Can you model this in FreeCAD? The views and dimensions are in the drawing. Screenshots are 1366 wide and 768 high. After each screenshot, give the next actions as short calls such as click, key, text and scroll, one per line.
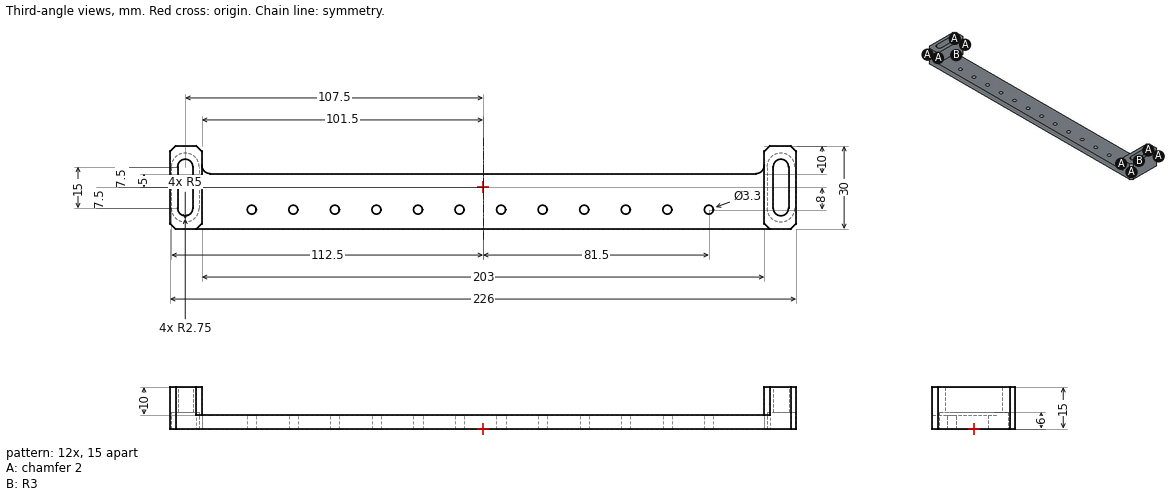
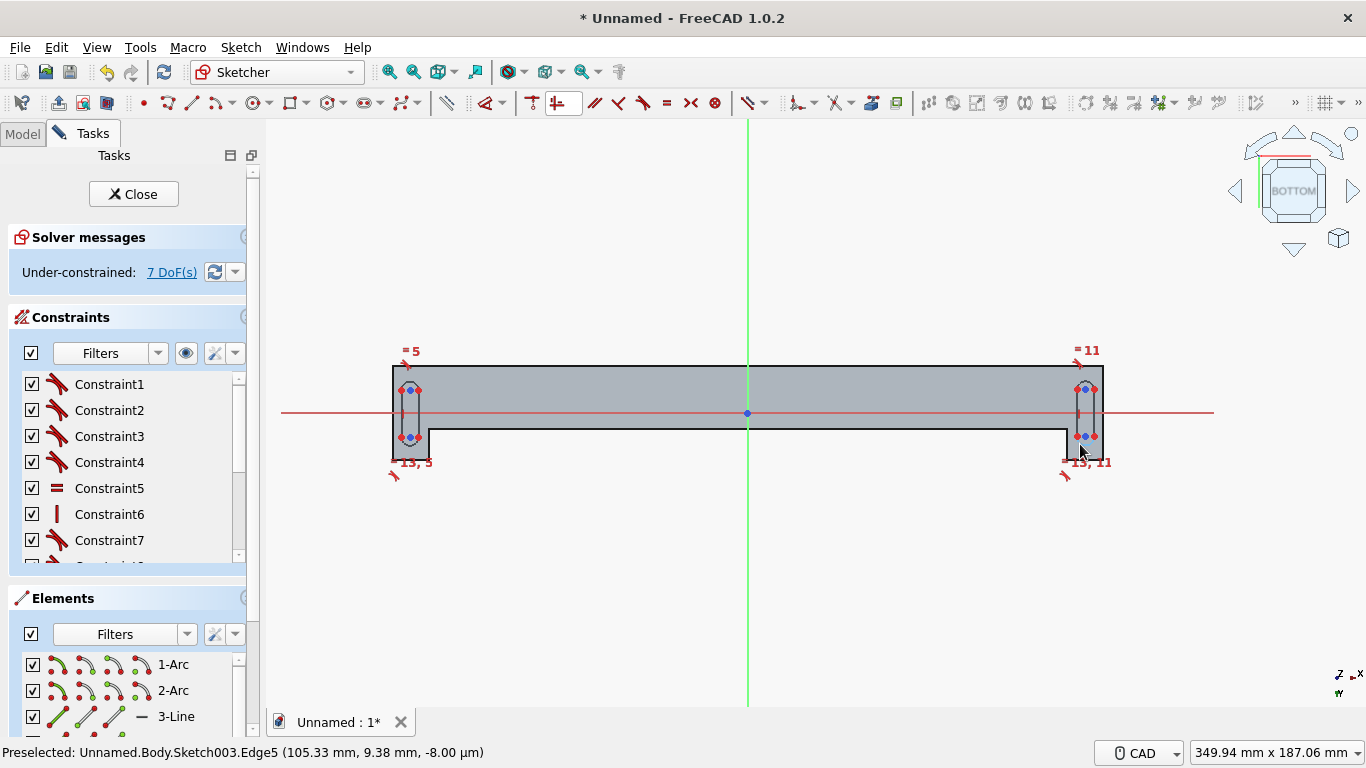
scroll(410, 437, up, 2)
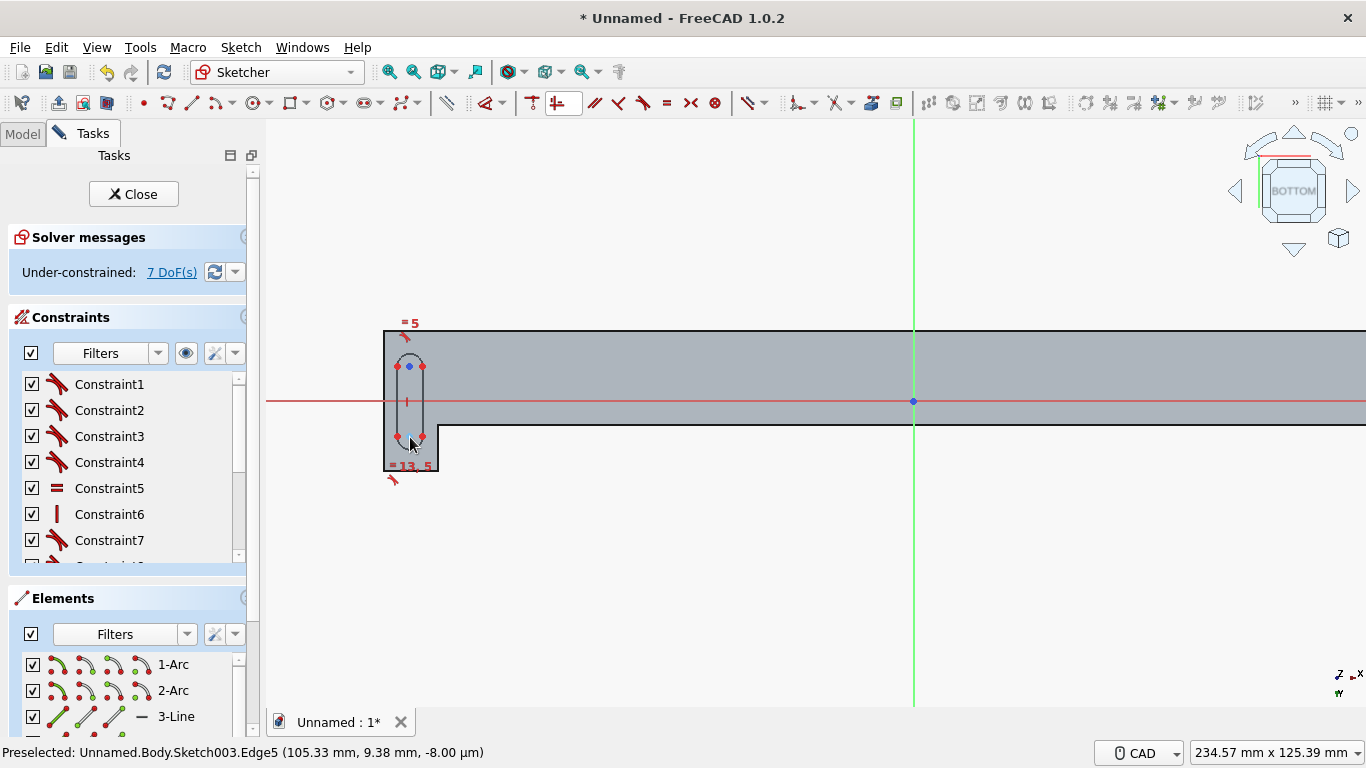
click(410, 437)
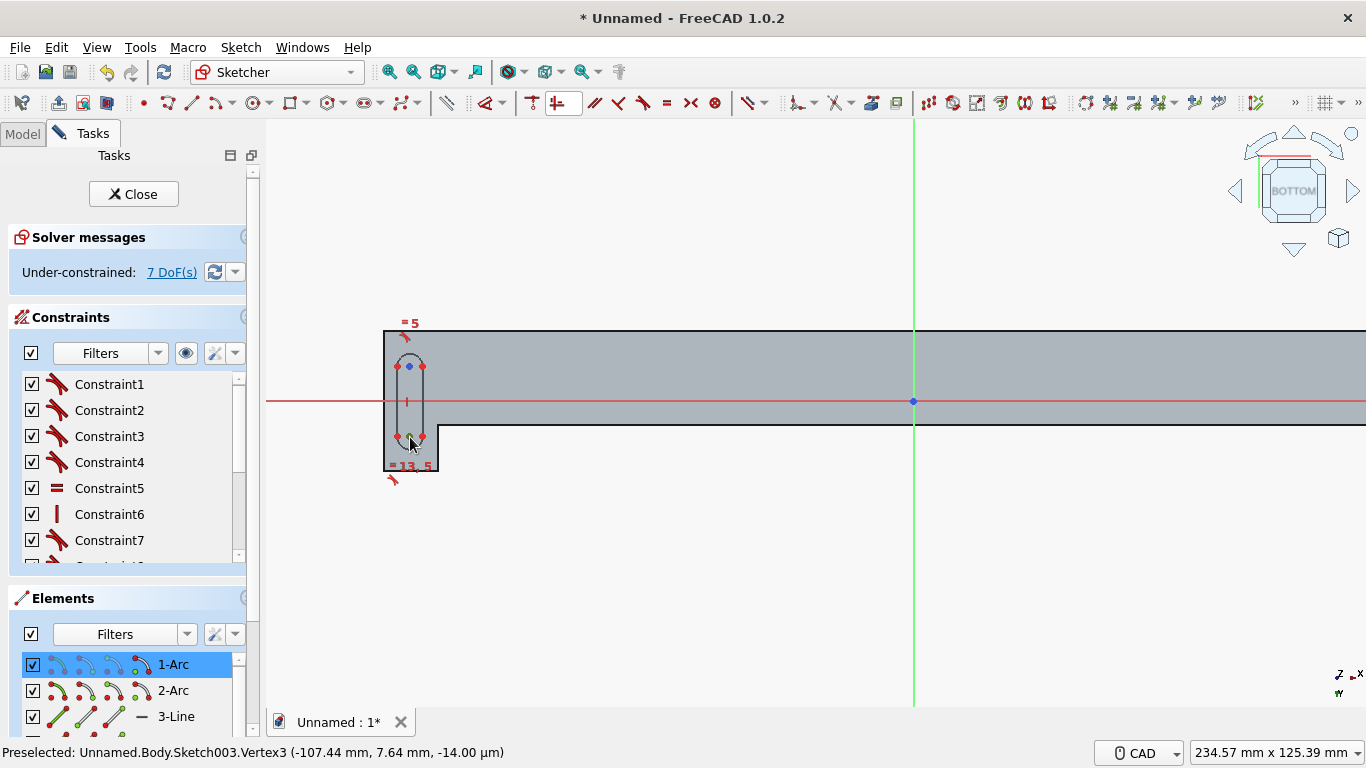
scroll(409, 437, down, 2)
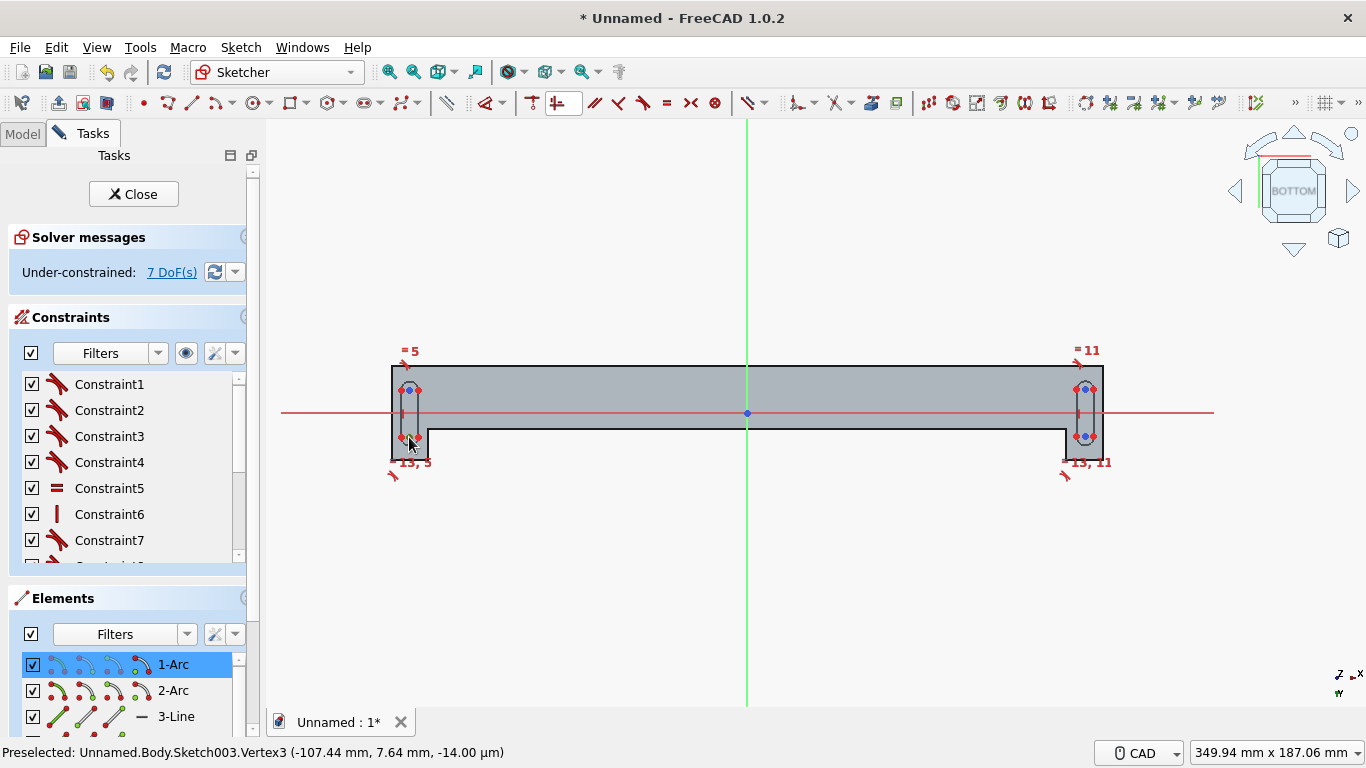
scroll(1085, 437, up, 2)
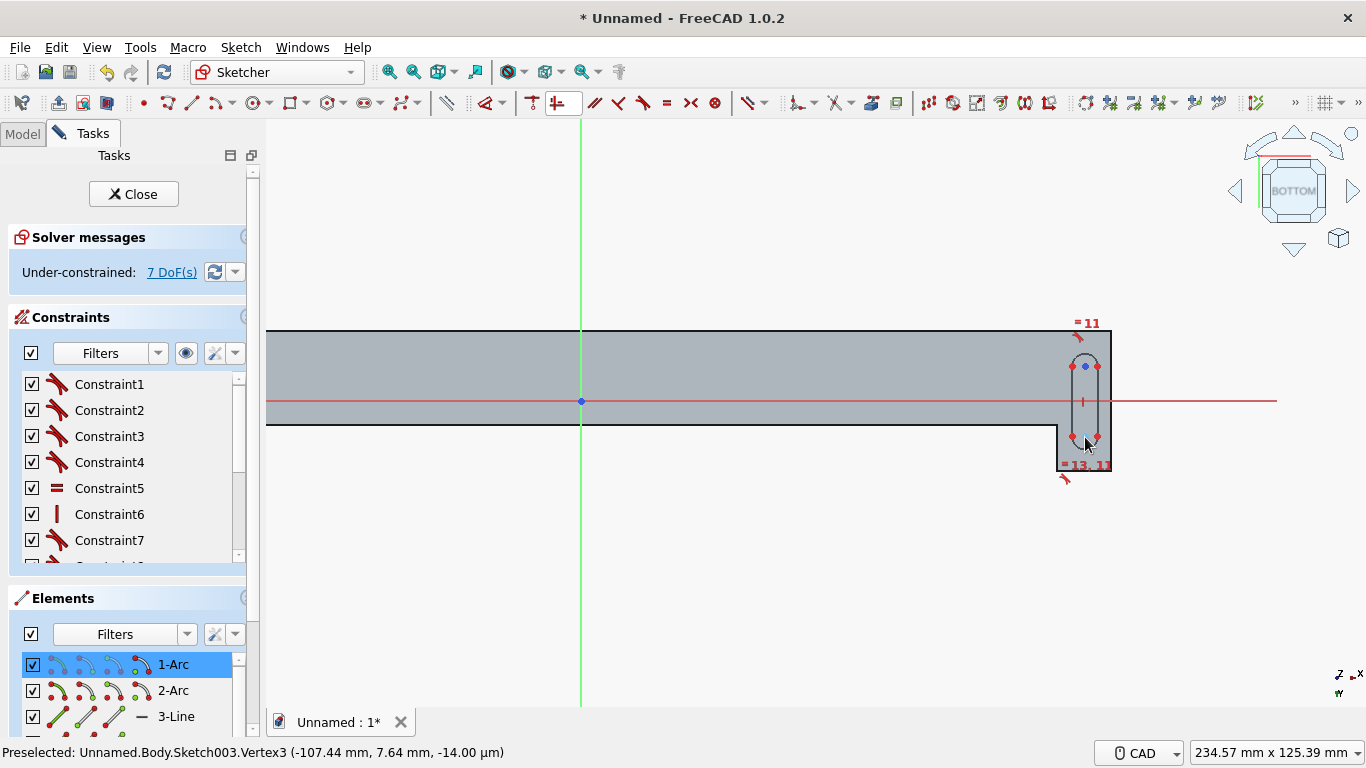
click(1085, 437)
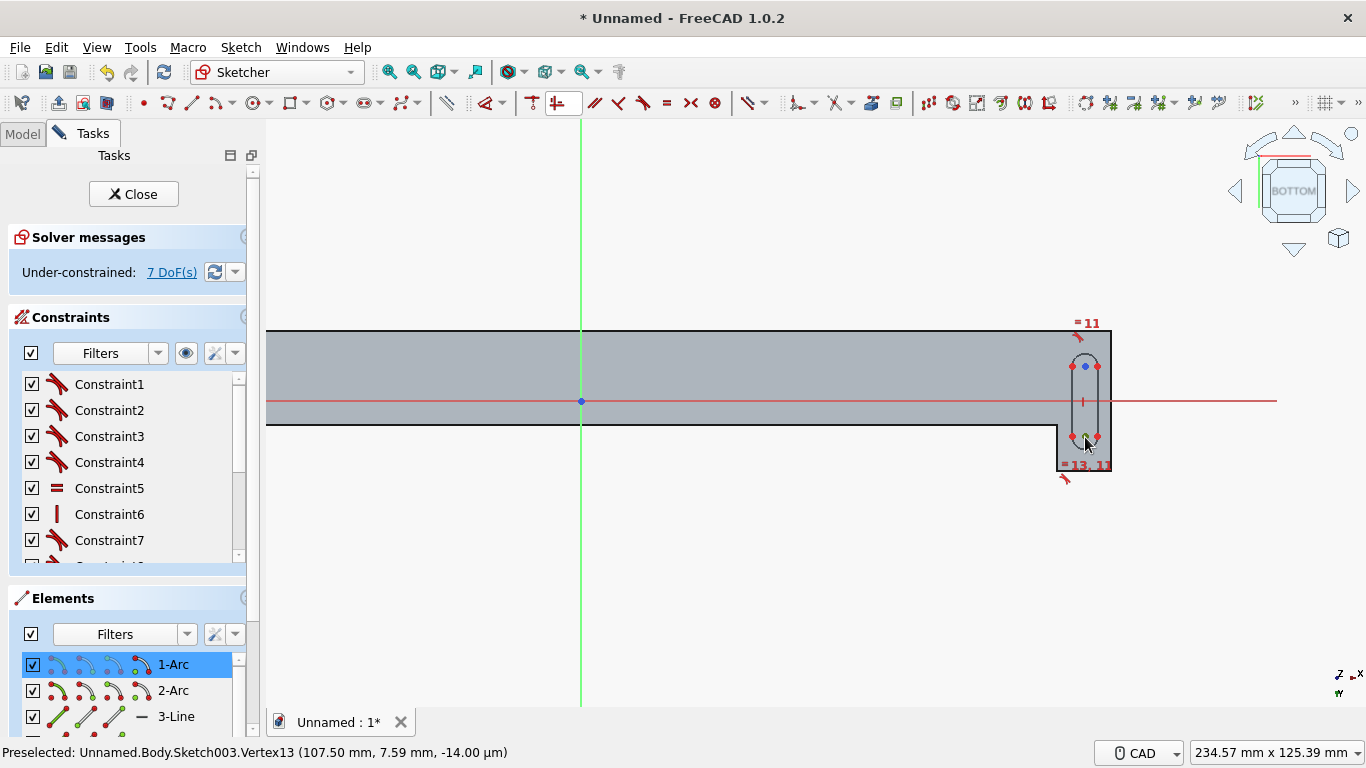
click(581, 641)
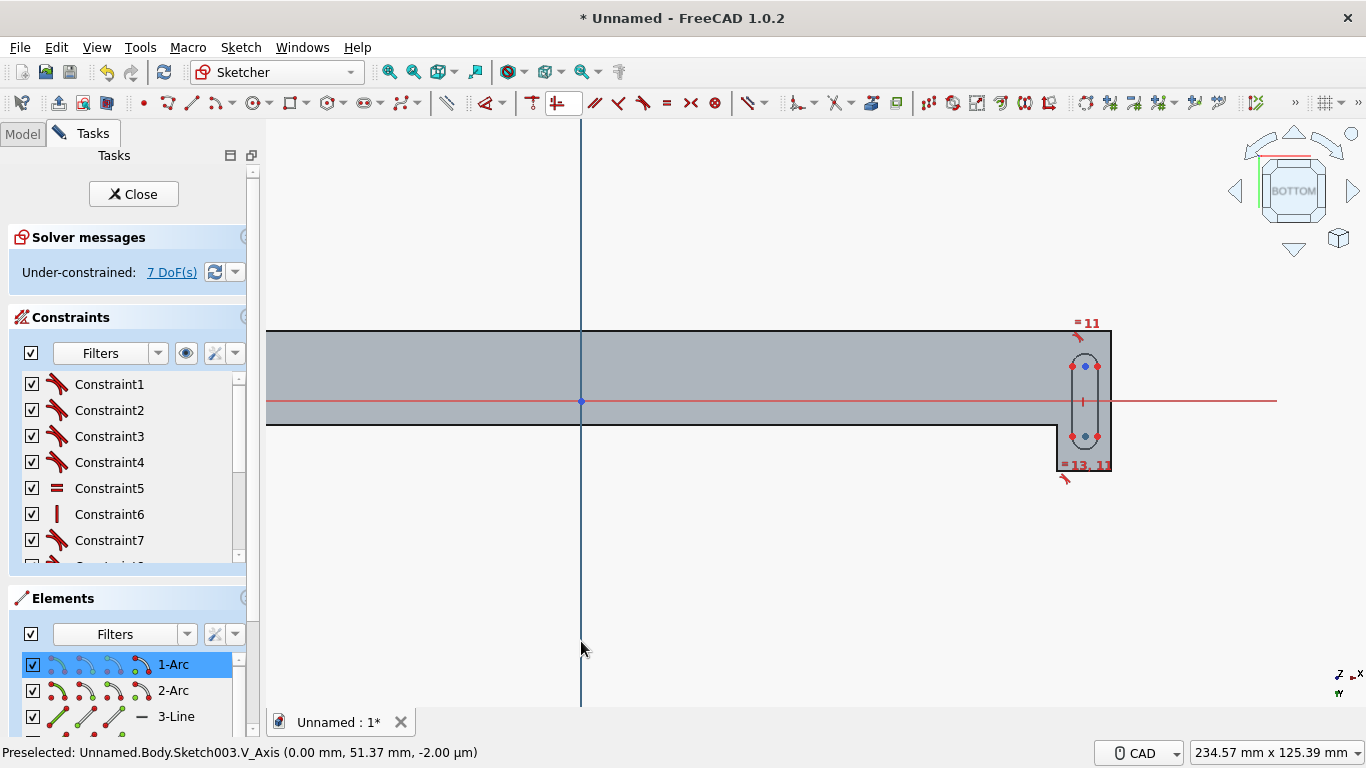
key(s)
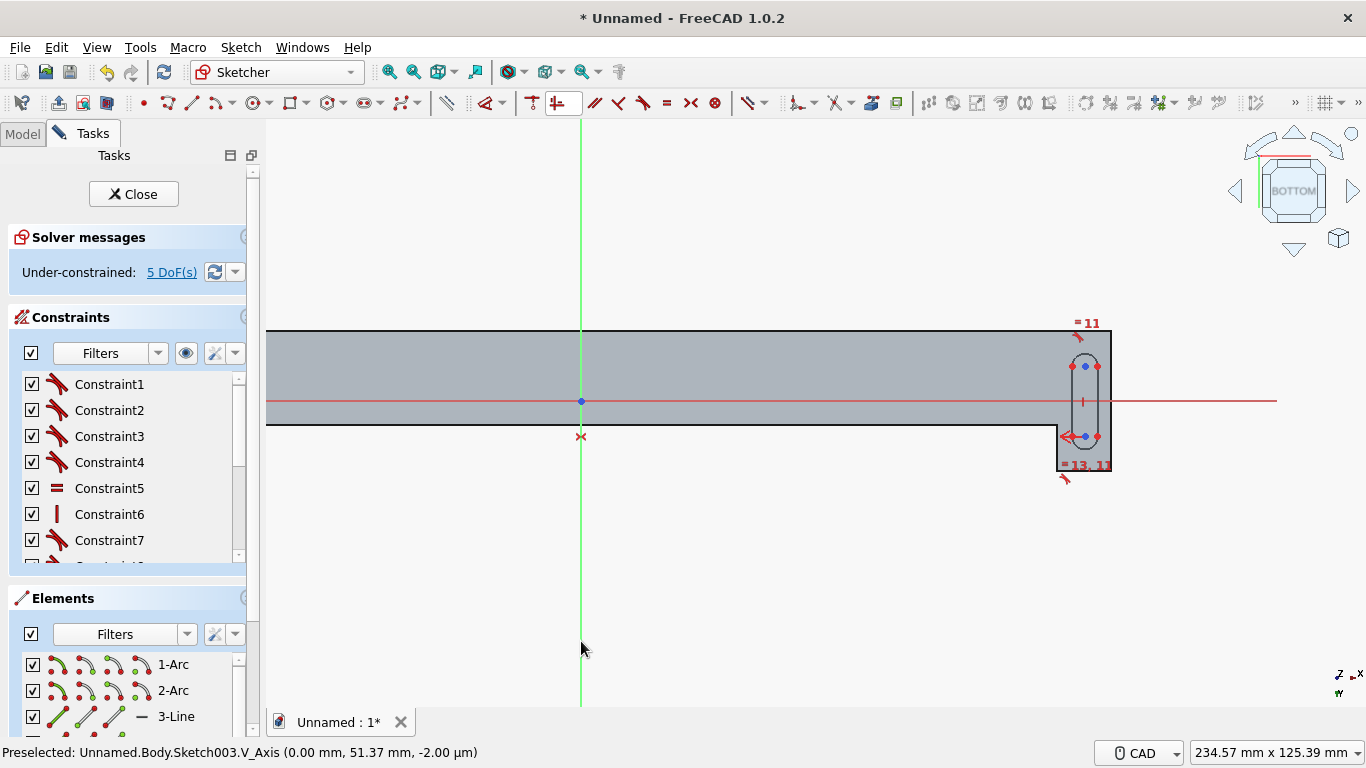
click(486, 104)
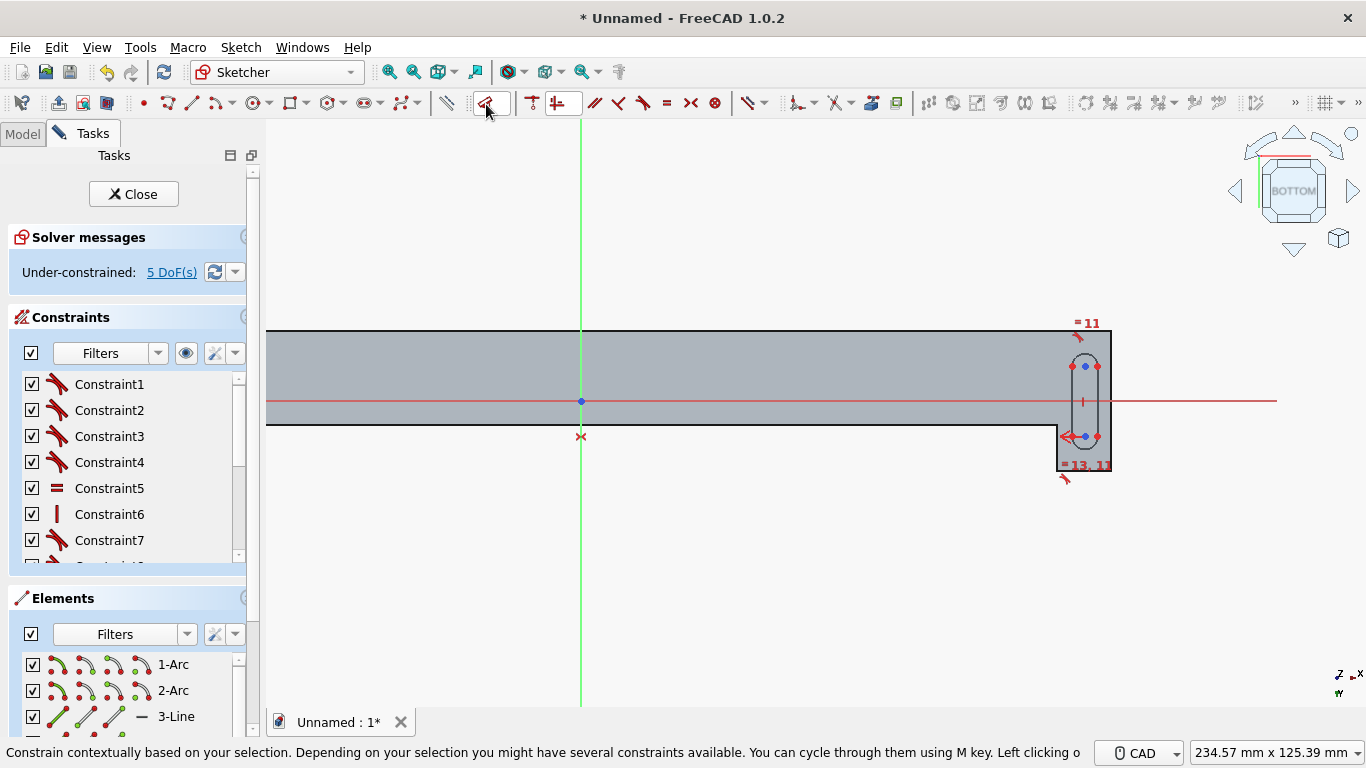
scroll(1086, 437, down, 2)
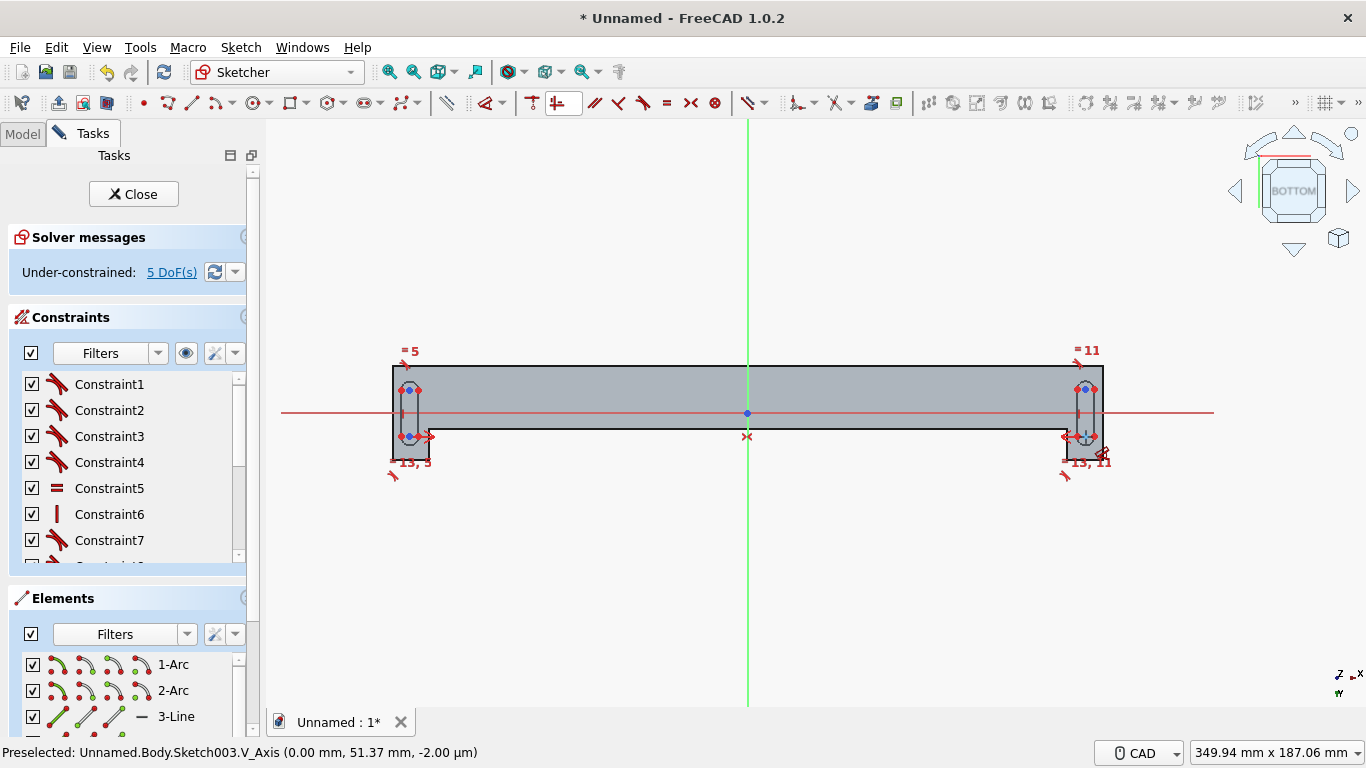
scroll(405, 444, up, 8)